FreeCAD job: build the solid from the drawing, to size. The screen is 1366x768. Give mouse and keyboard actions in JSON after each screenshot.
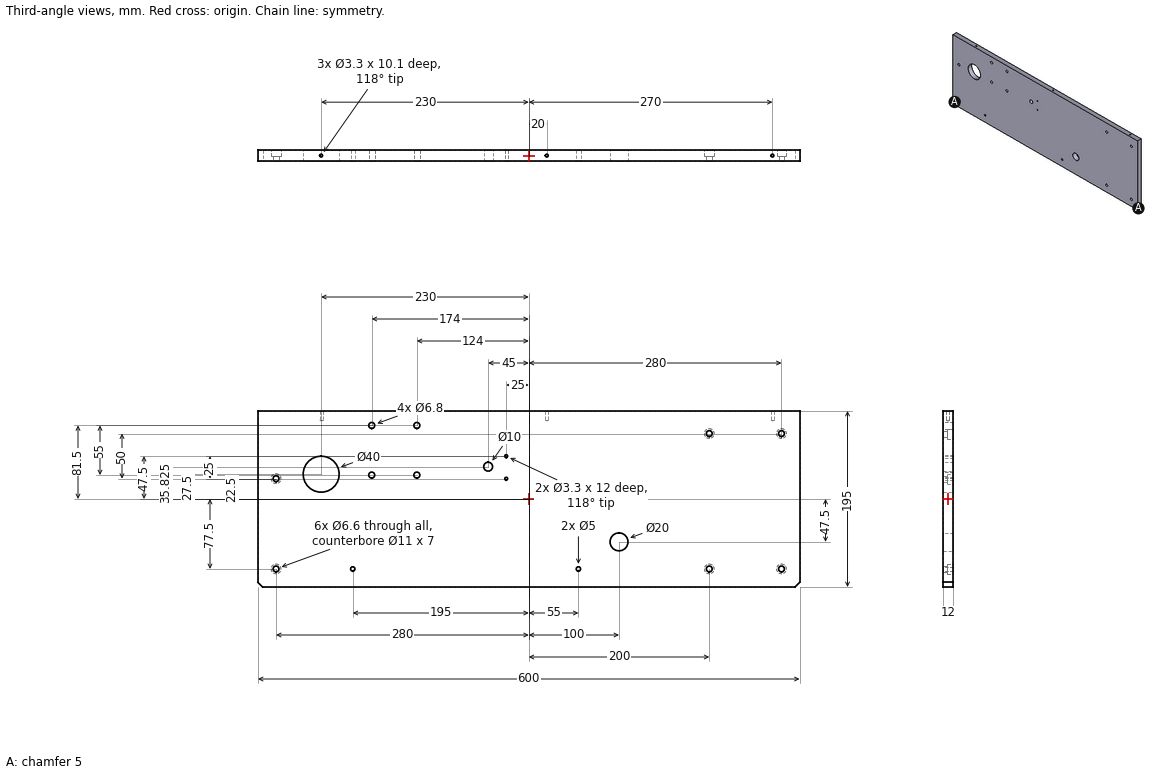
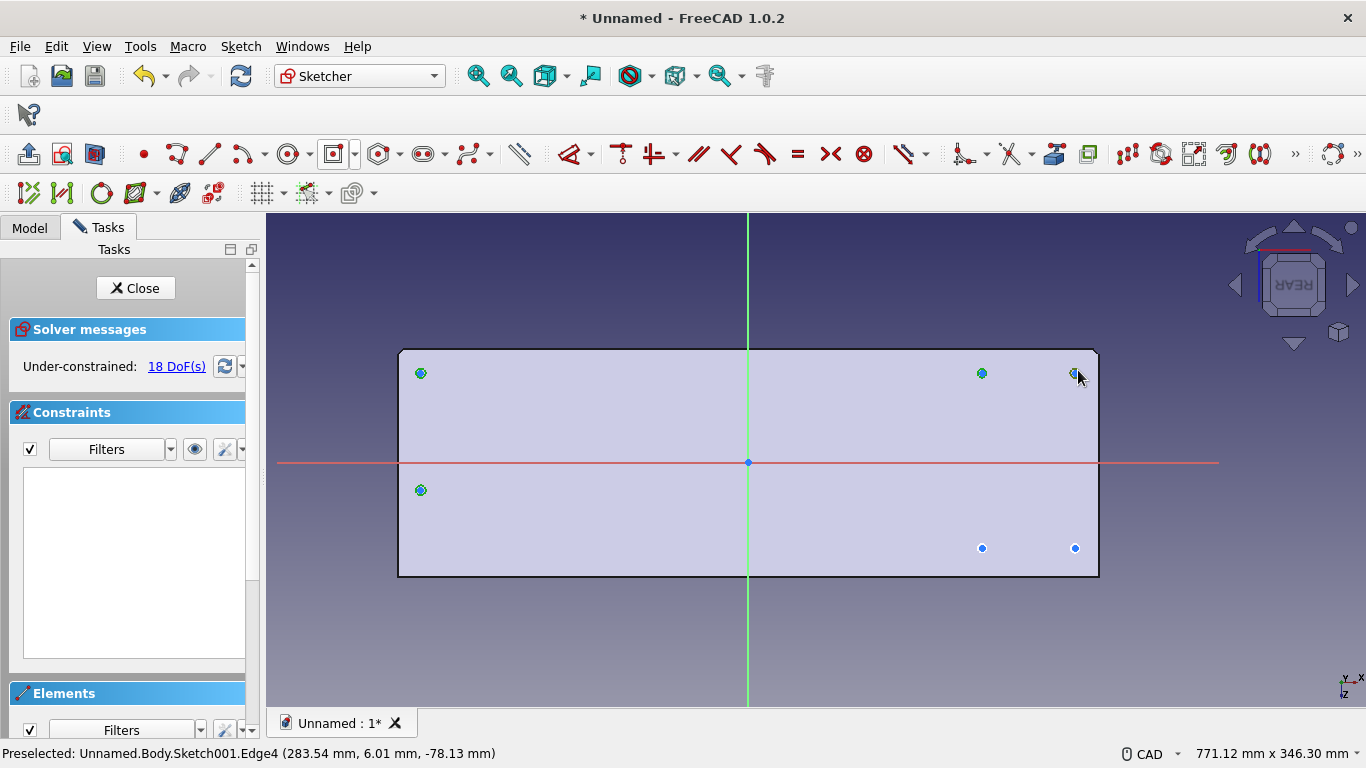
{"action": "scroll", "coordinate": [1078, 545], "scroll_direction": "up", "scroll_amount": 6}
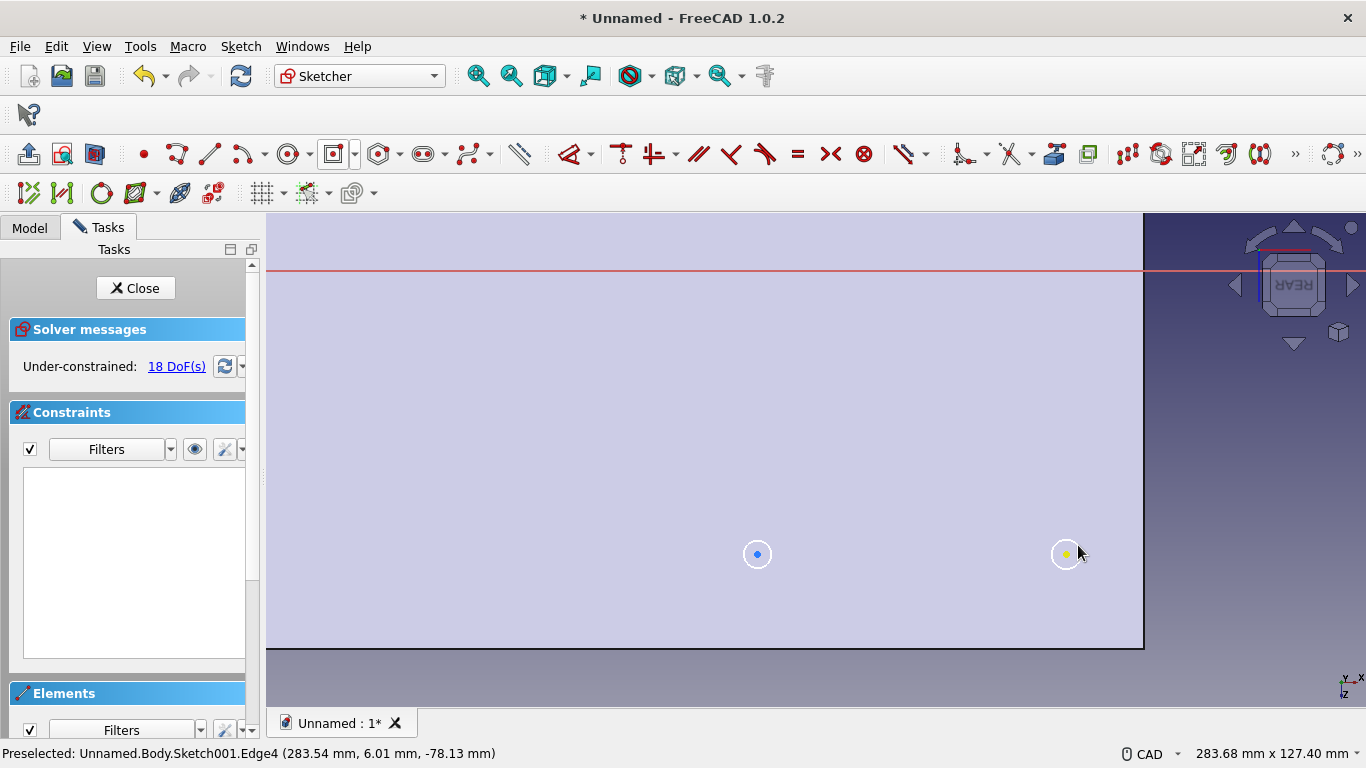
{"action": "left_click", "coordinate": [1077, 544]}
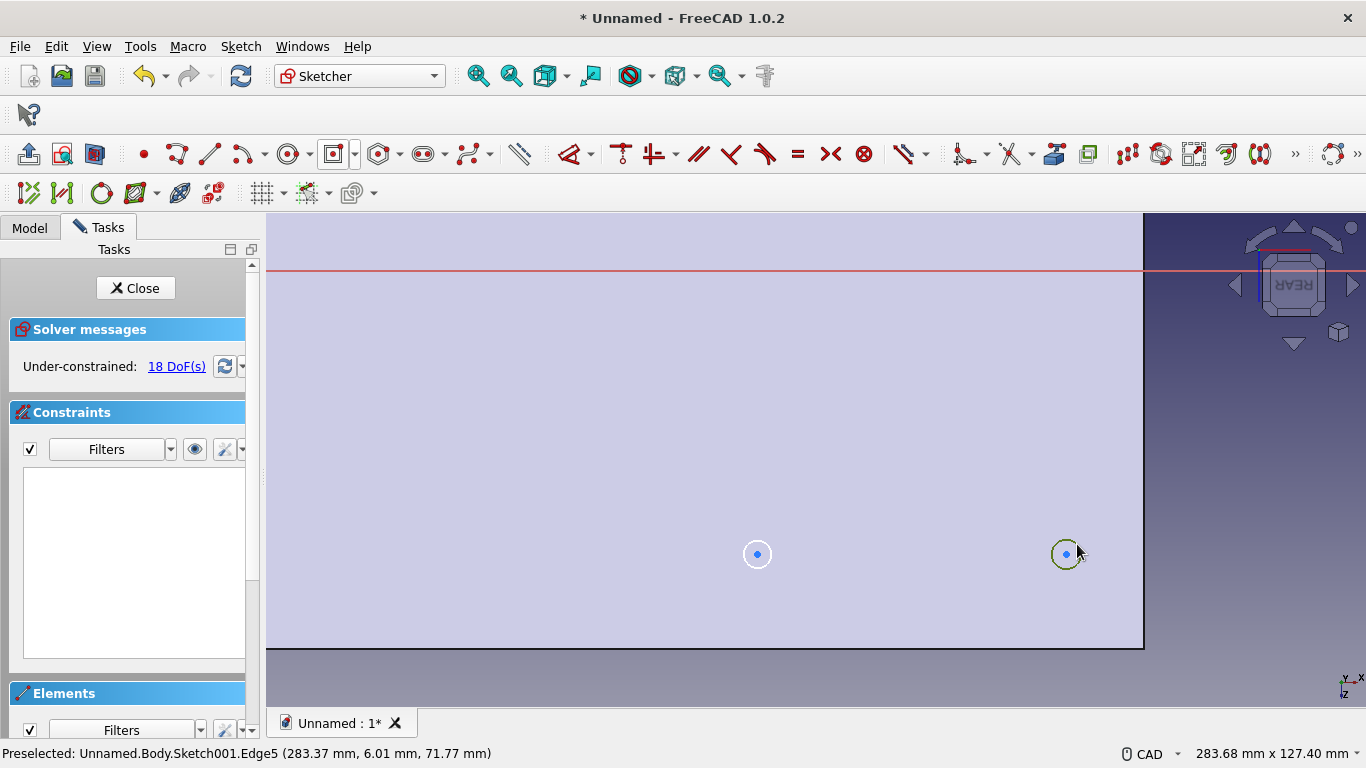
{"action": "left_click", "coordinate": [767, 545]}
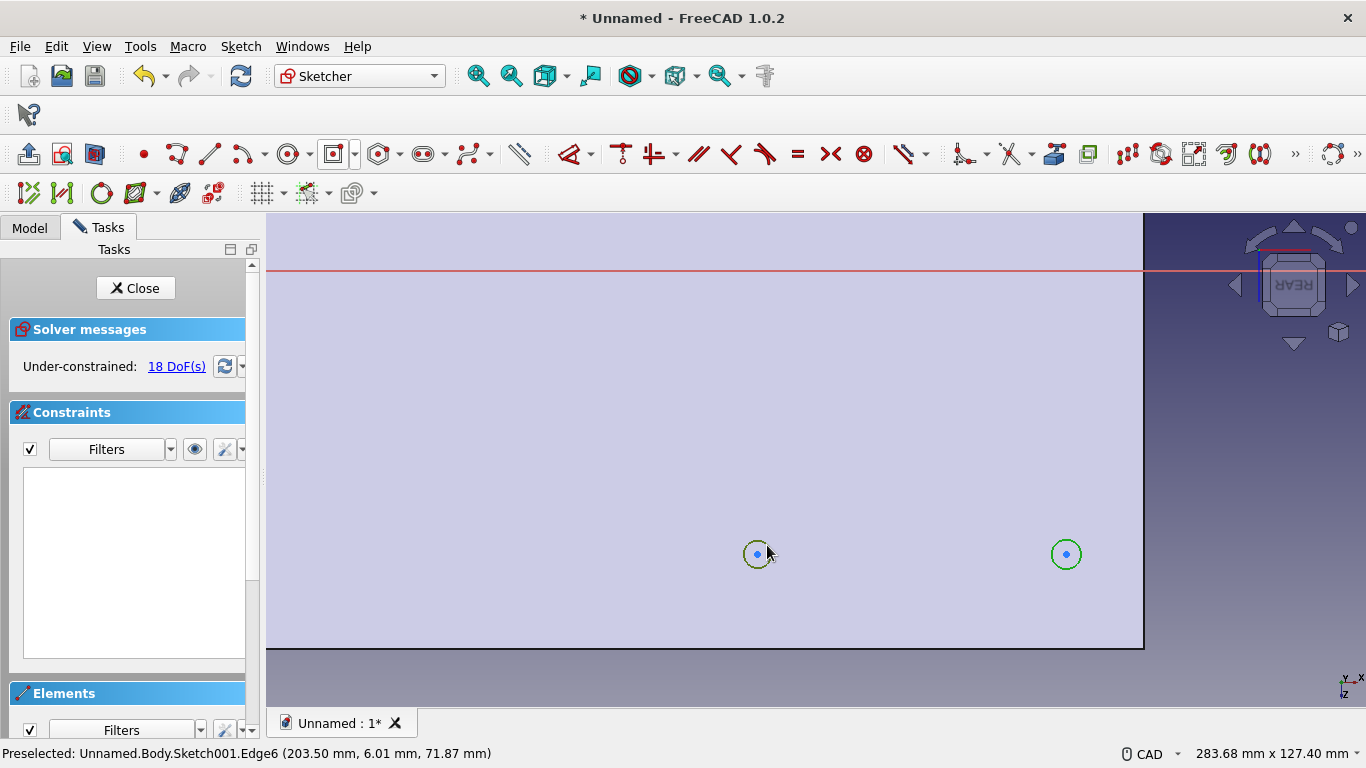
{"action": "left_click", "coordinate": [798, 154]}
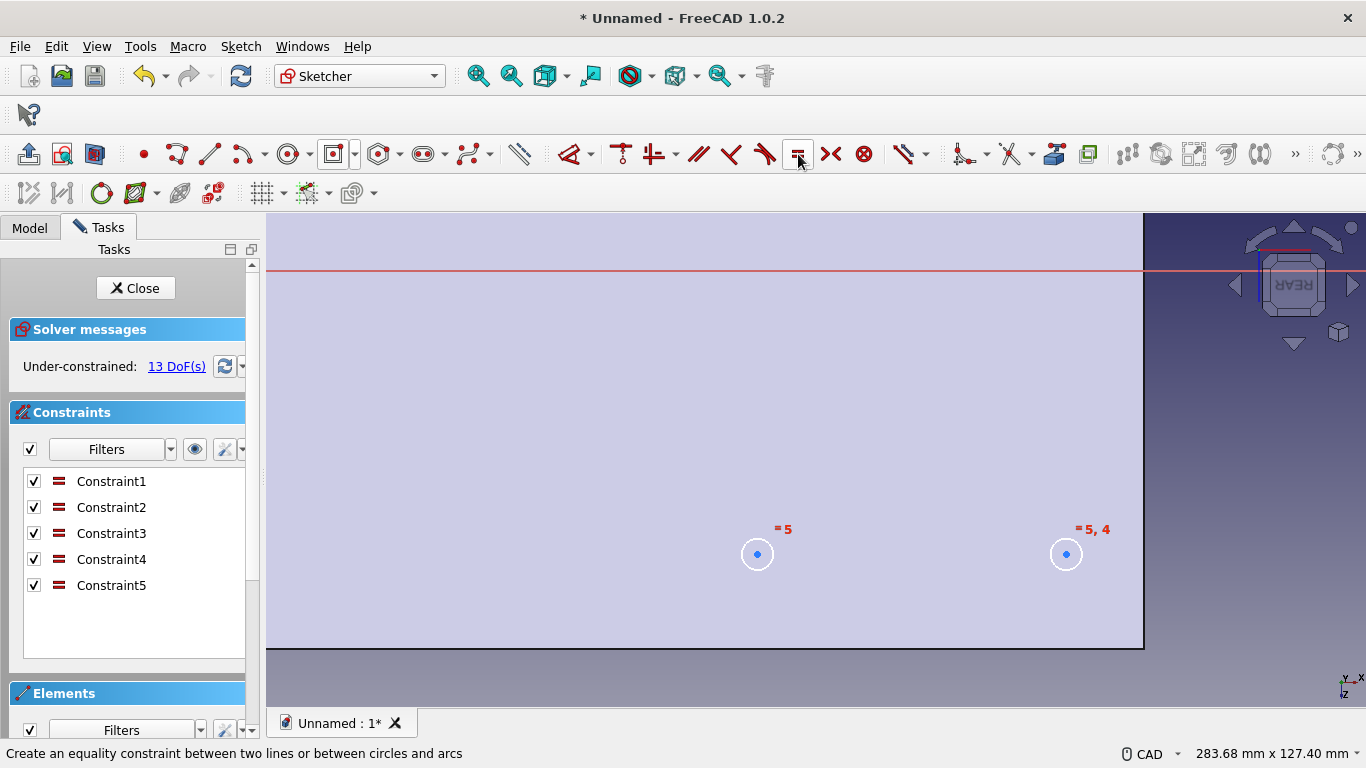
{"action": "scroll", "coordinate": [1078, 546], "scroll_direction": "down", "scroll_amount": 6}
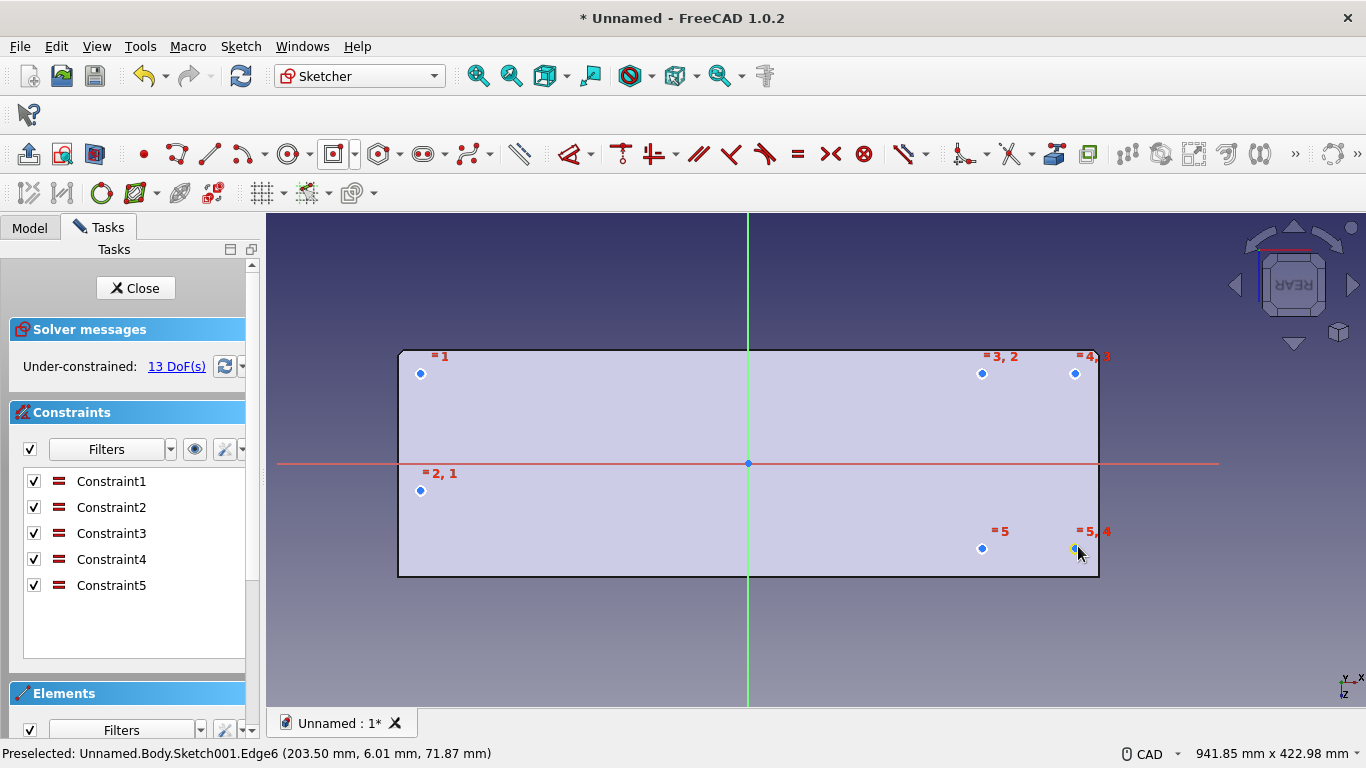
{"action": "left_click", "coordinate": [421, 374]}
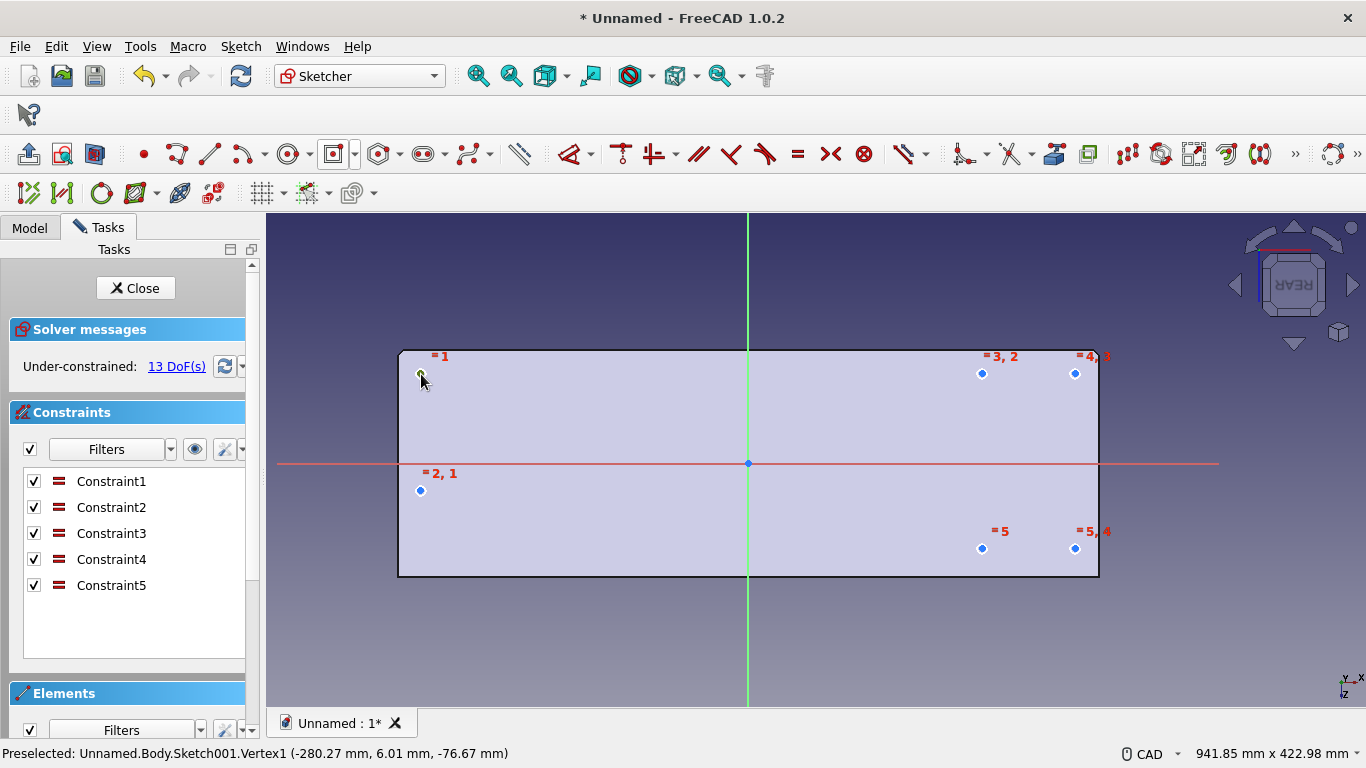
{"action": "left_click", "coordinate": [1075, 374]}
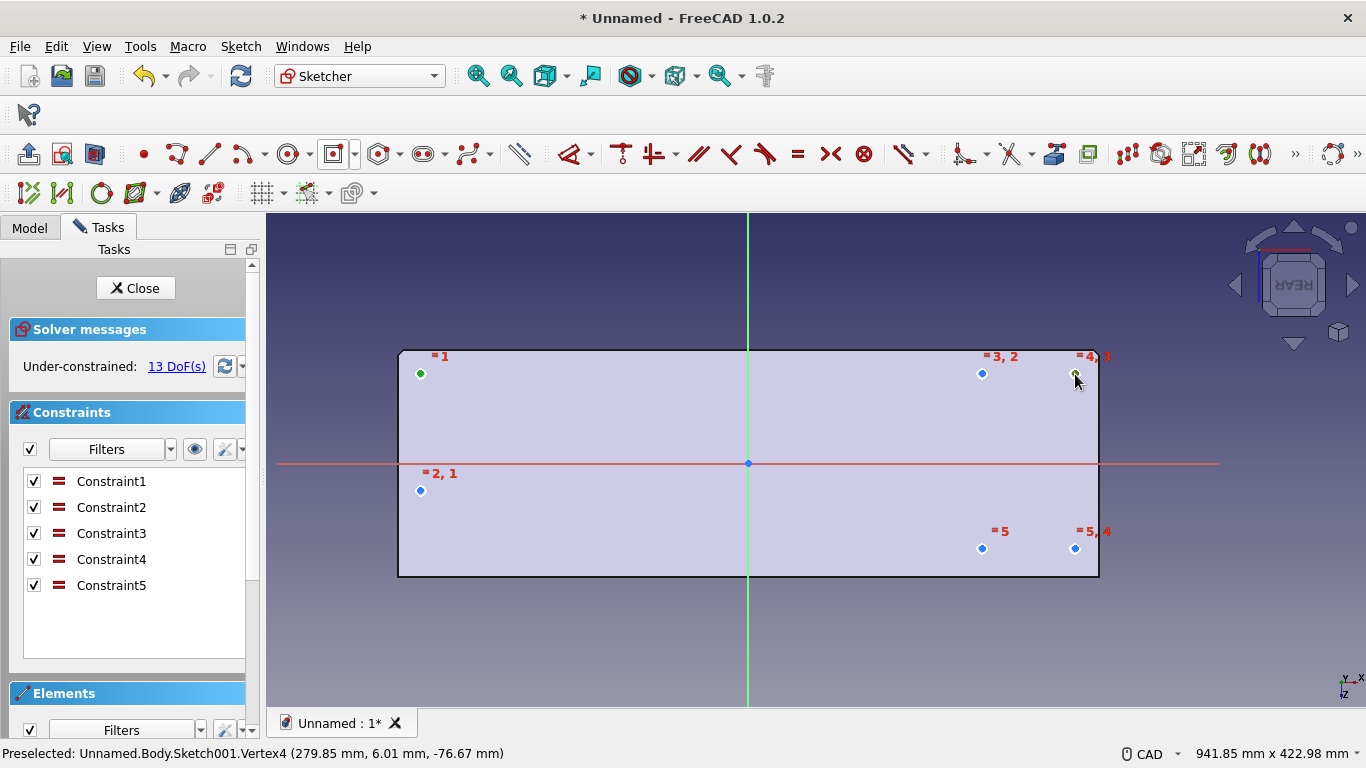
{"action": "left_click", "coordinate": [748, 648]}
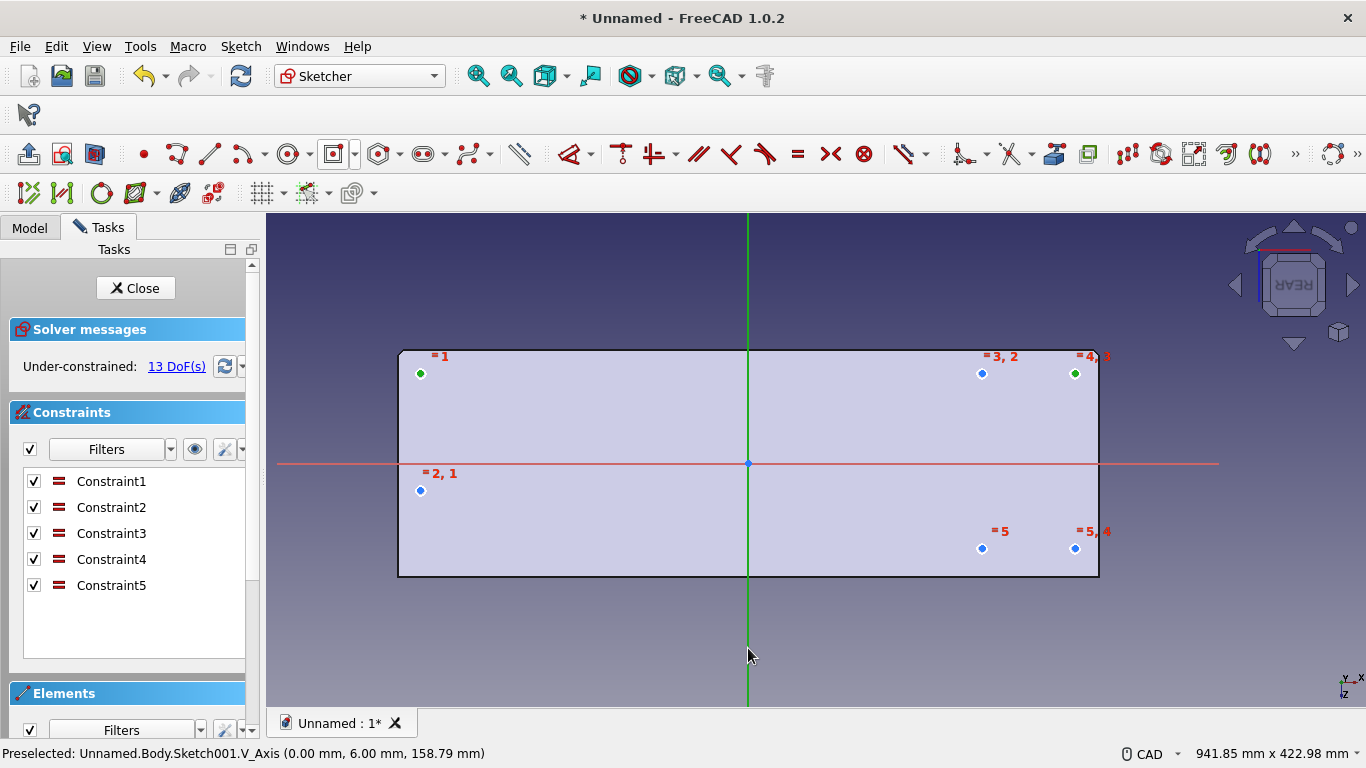
{"action": "left_click", "coordinate": [831, 154]}